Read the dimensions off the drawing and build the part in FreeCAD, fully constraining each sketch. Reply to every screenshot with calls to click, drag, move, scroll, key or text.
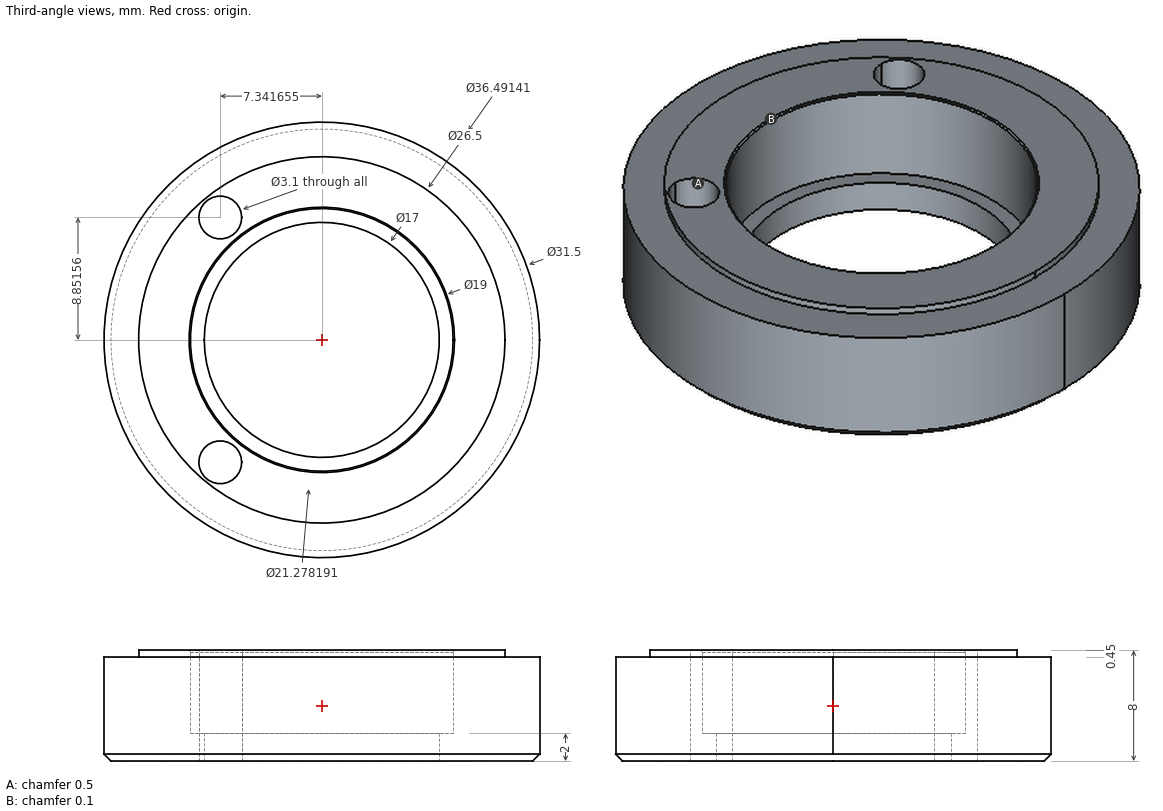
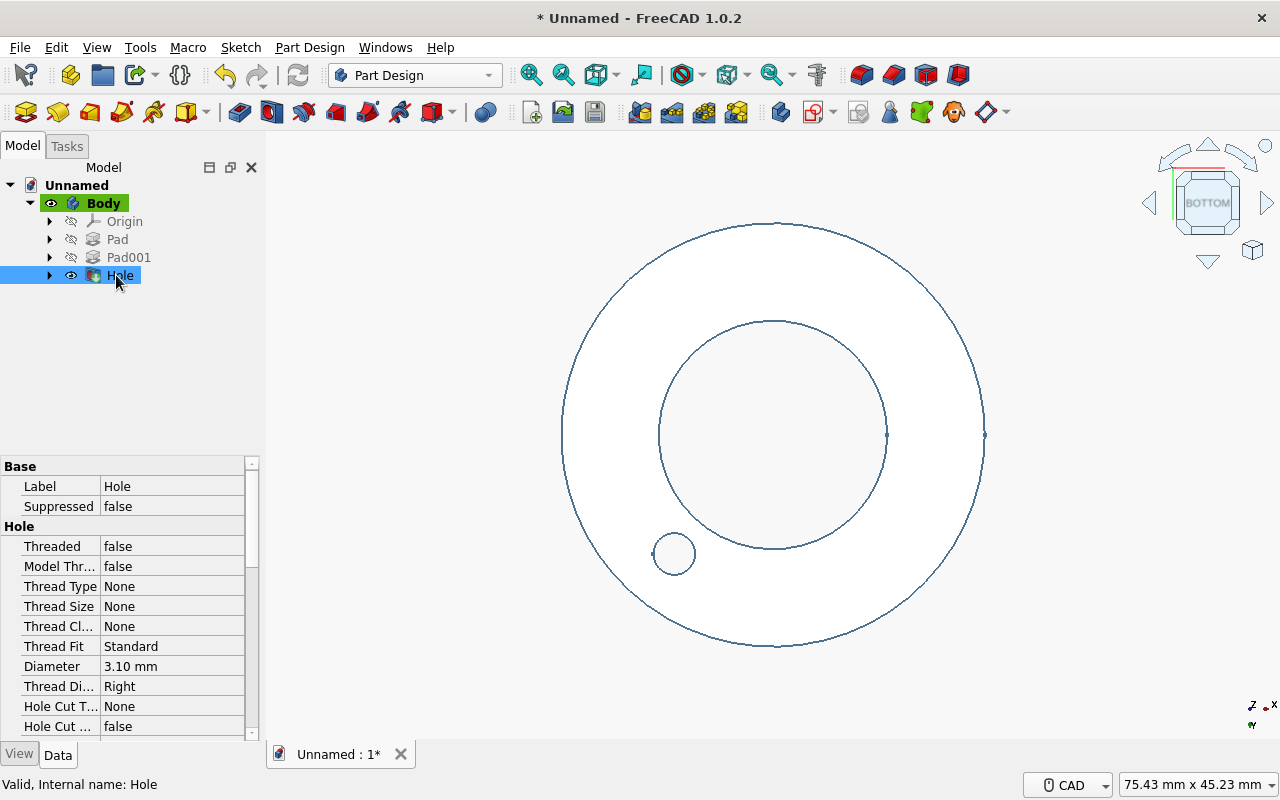
click(640, 112)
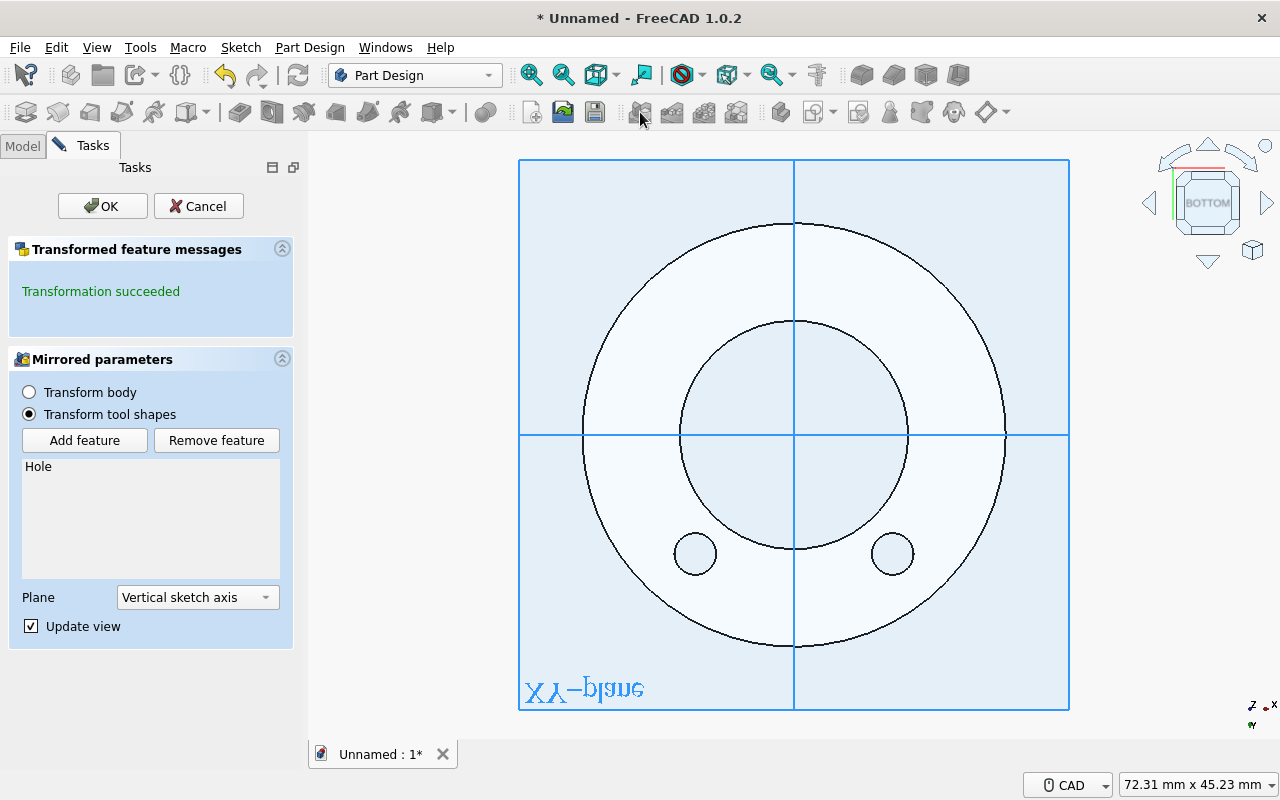
click(198, 598)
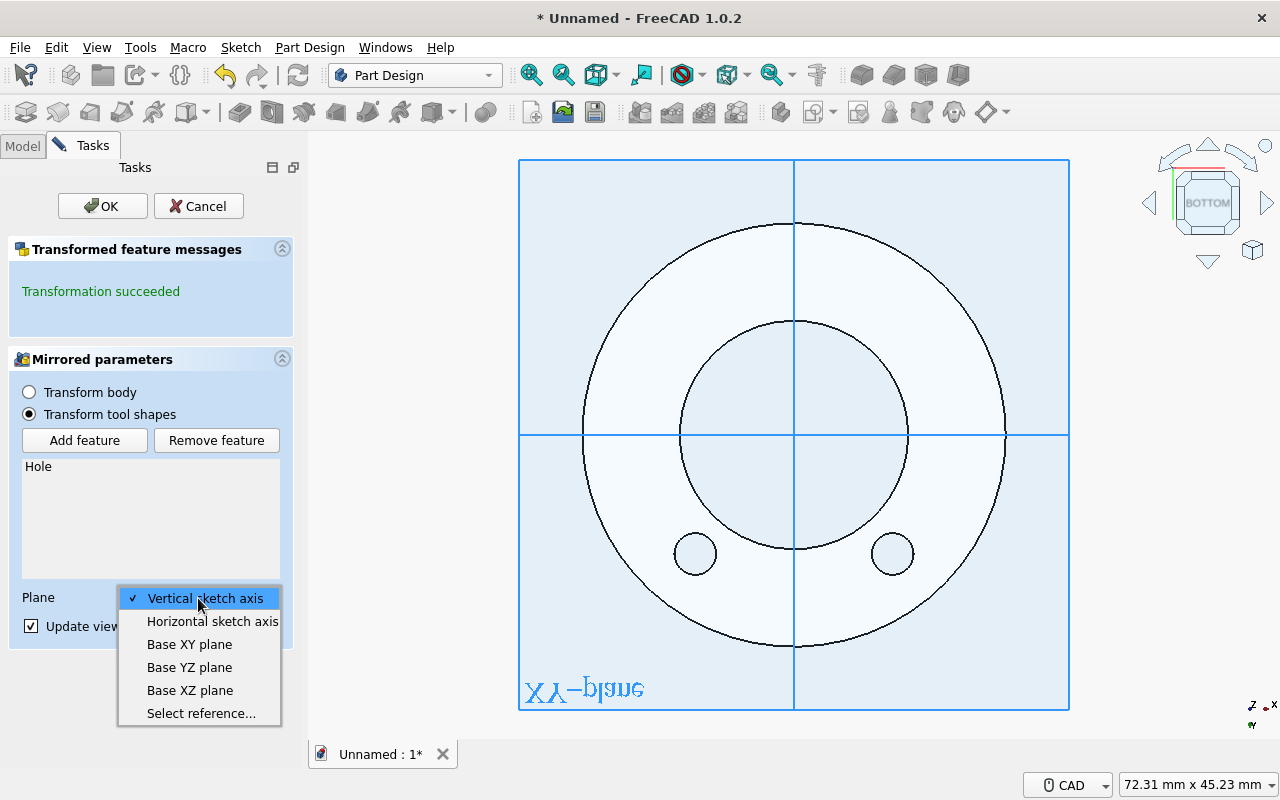
click(198, 690)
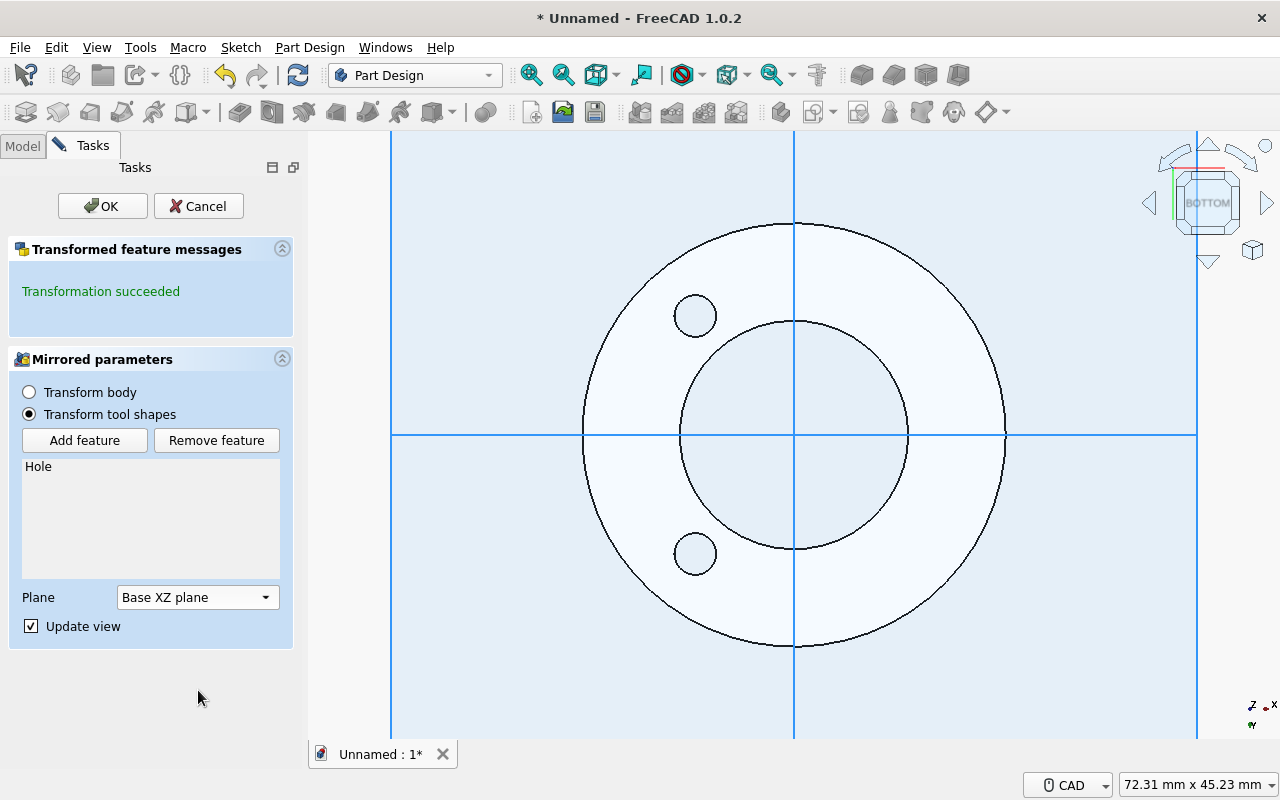
click(103, 206)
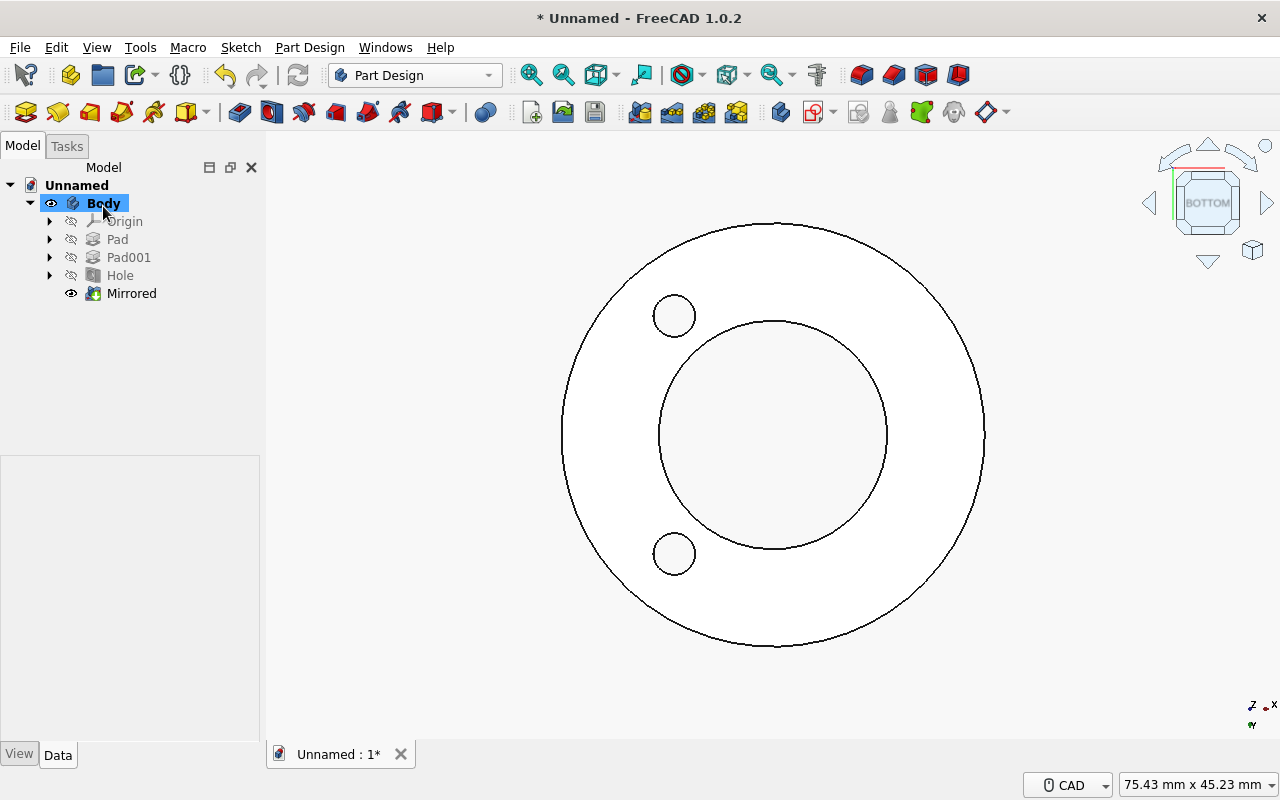
key(0)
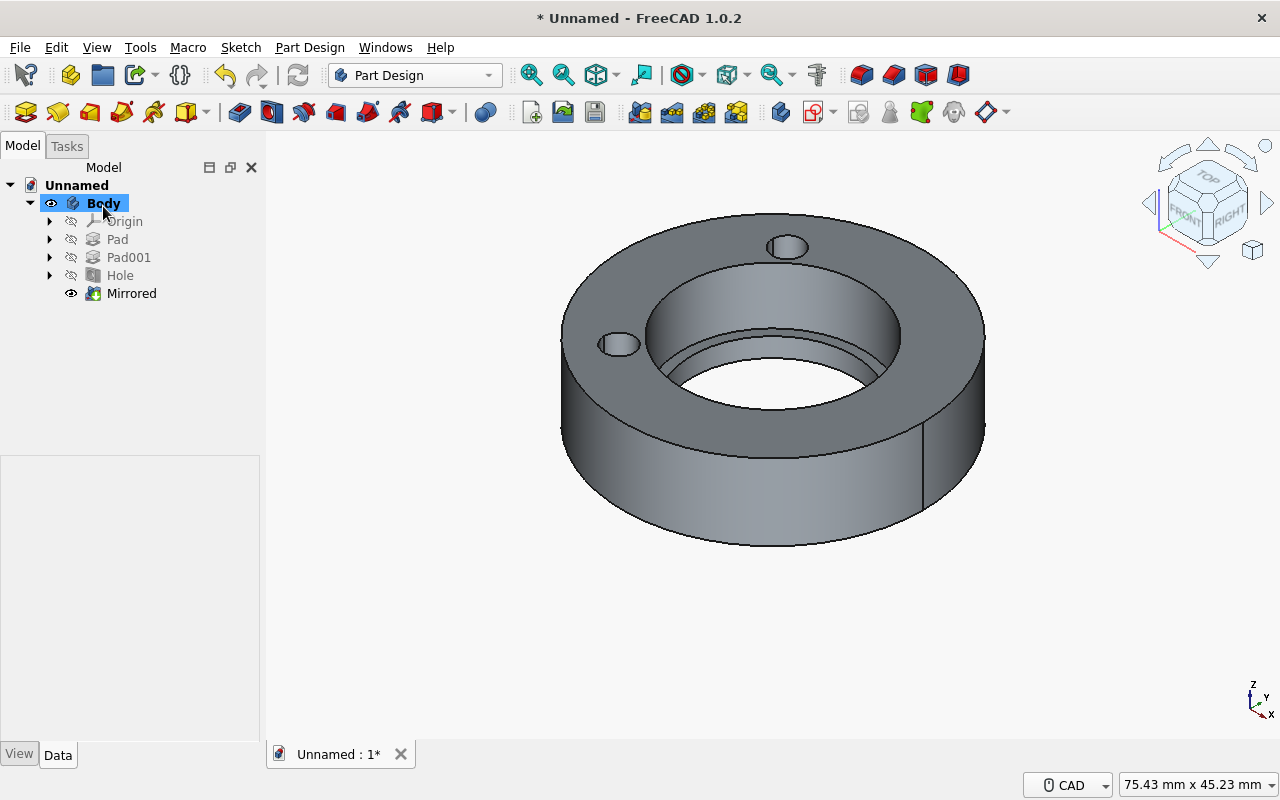
click(944, 335)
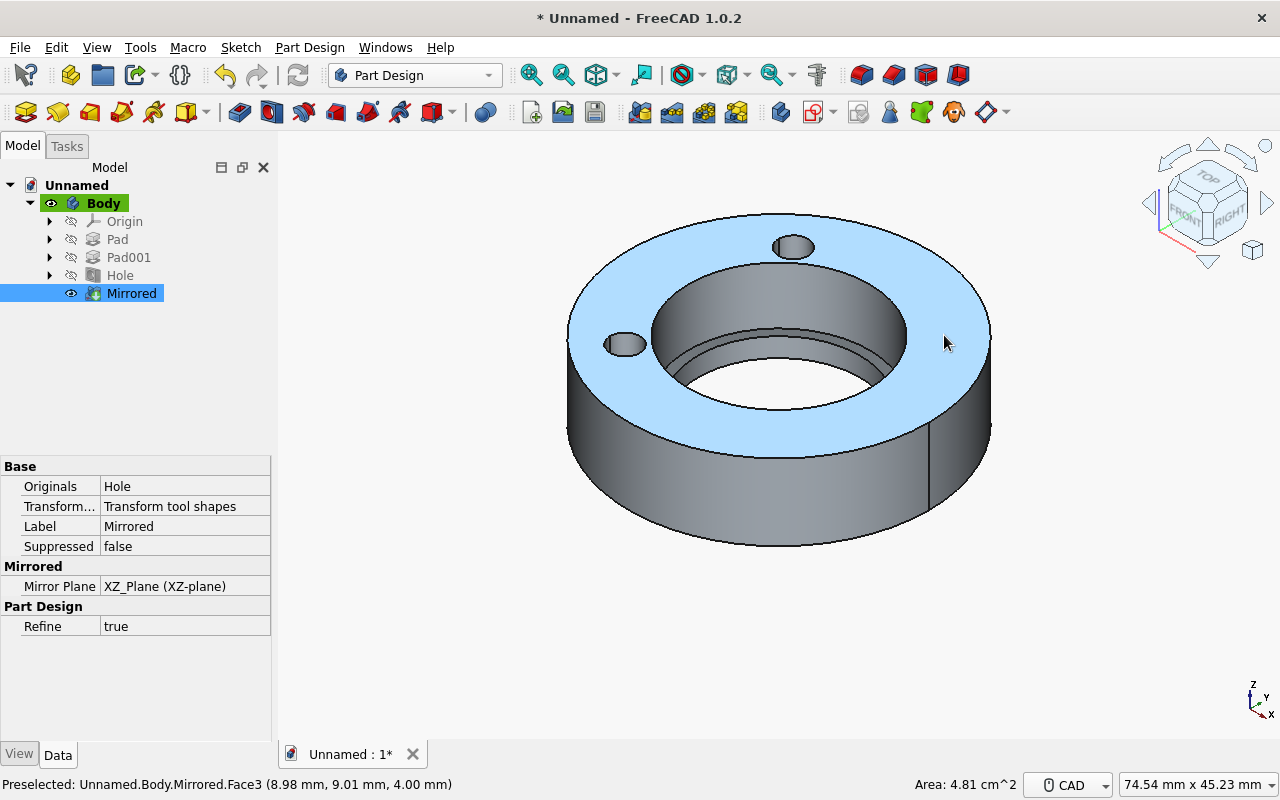
click(814, 112)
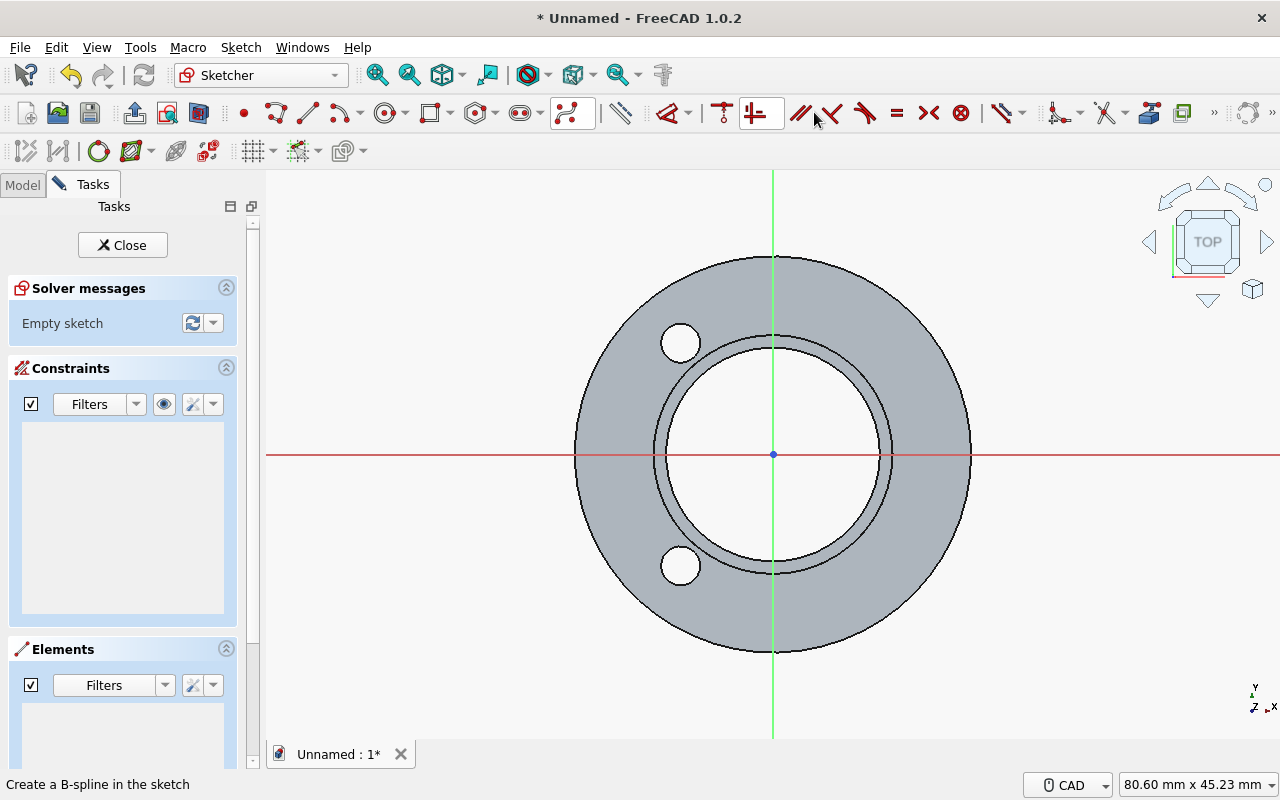
click(386, 114)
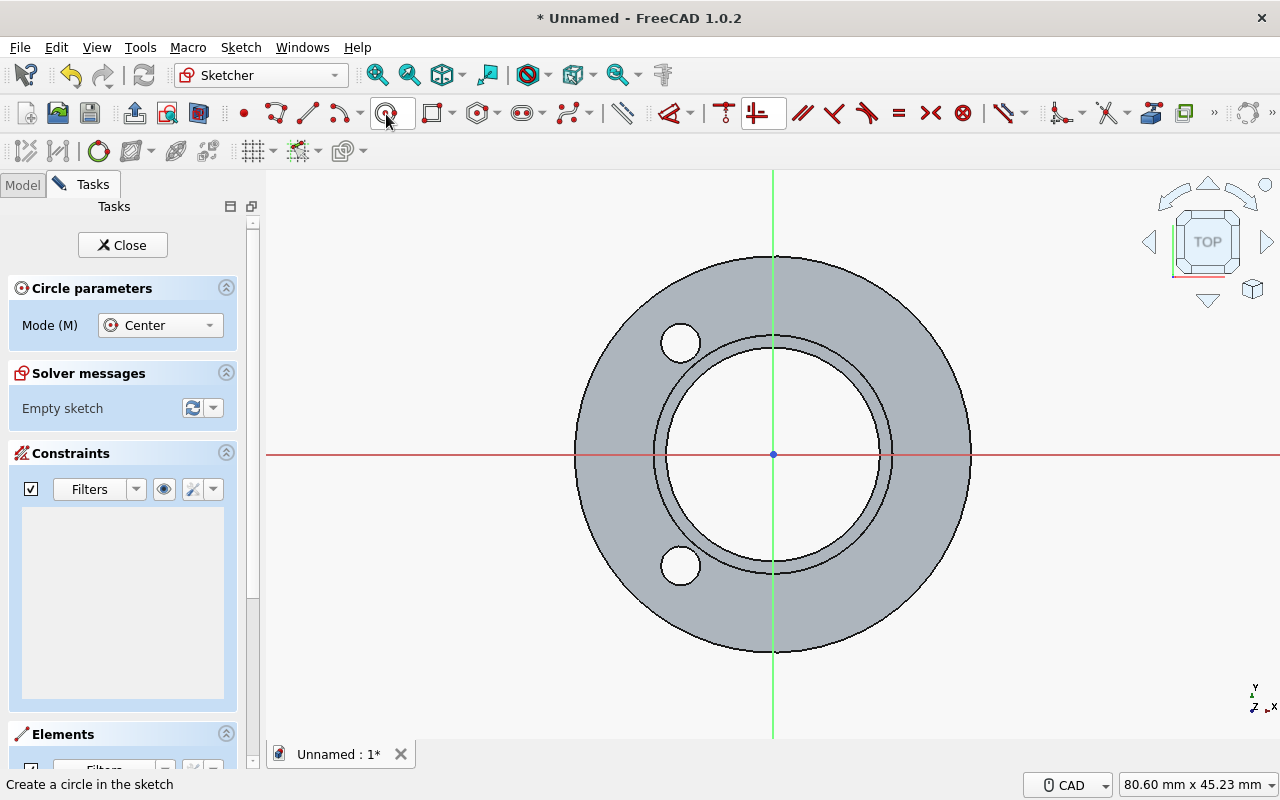
click(773, 454)
move(935, 292)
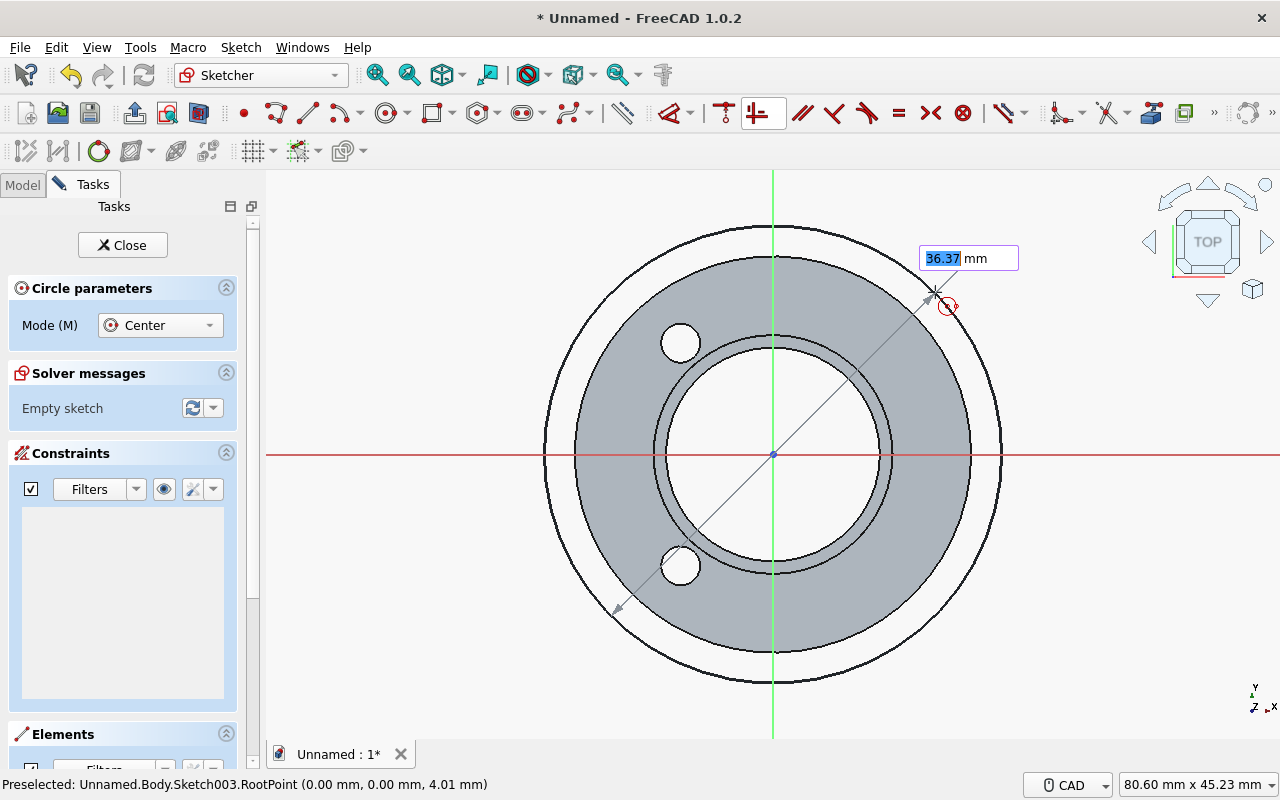
text(36.49141)
key(Return)